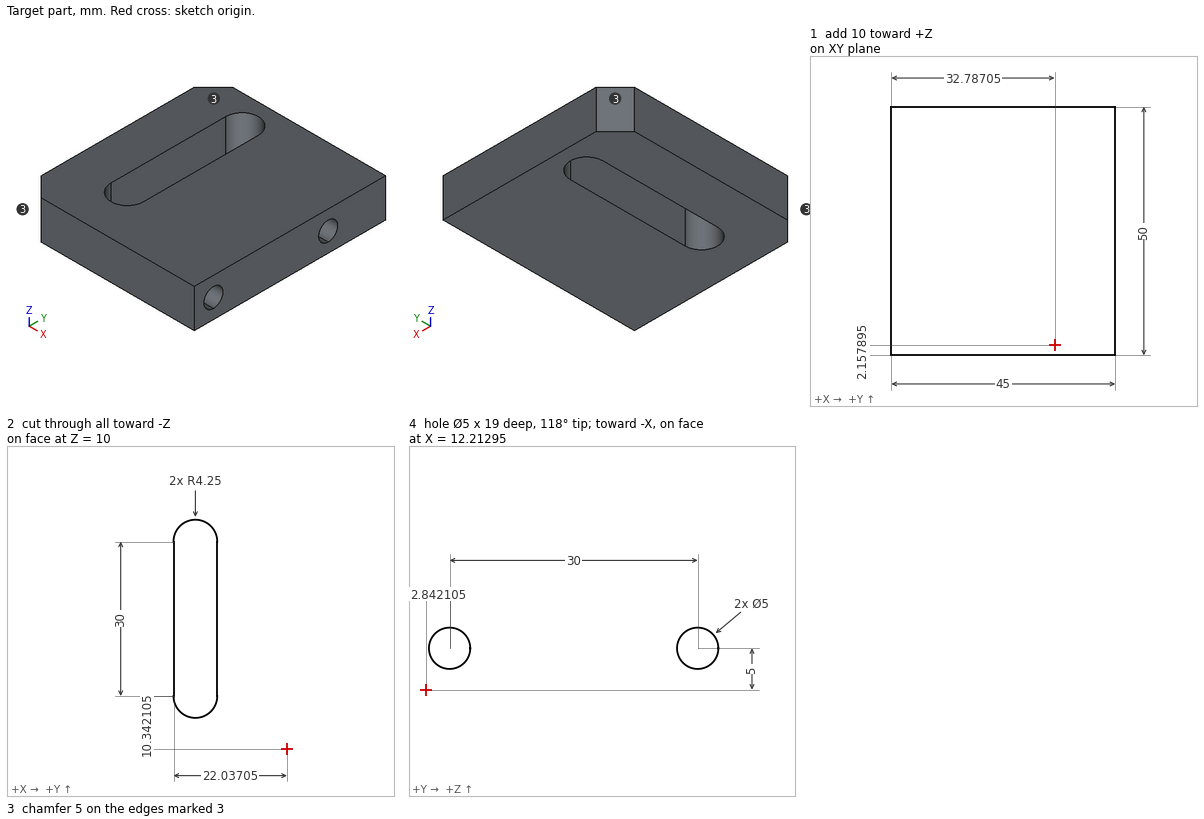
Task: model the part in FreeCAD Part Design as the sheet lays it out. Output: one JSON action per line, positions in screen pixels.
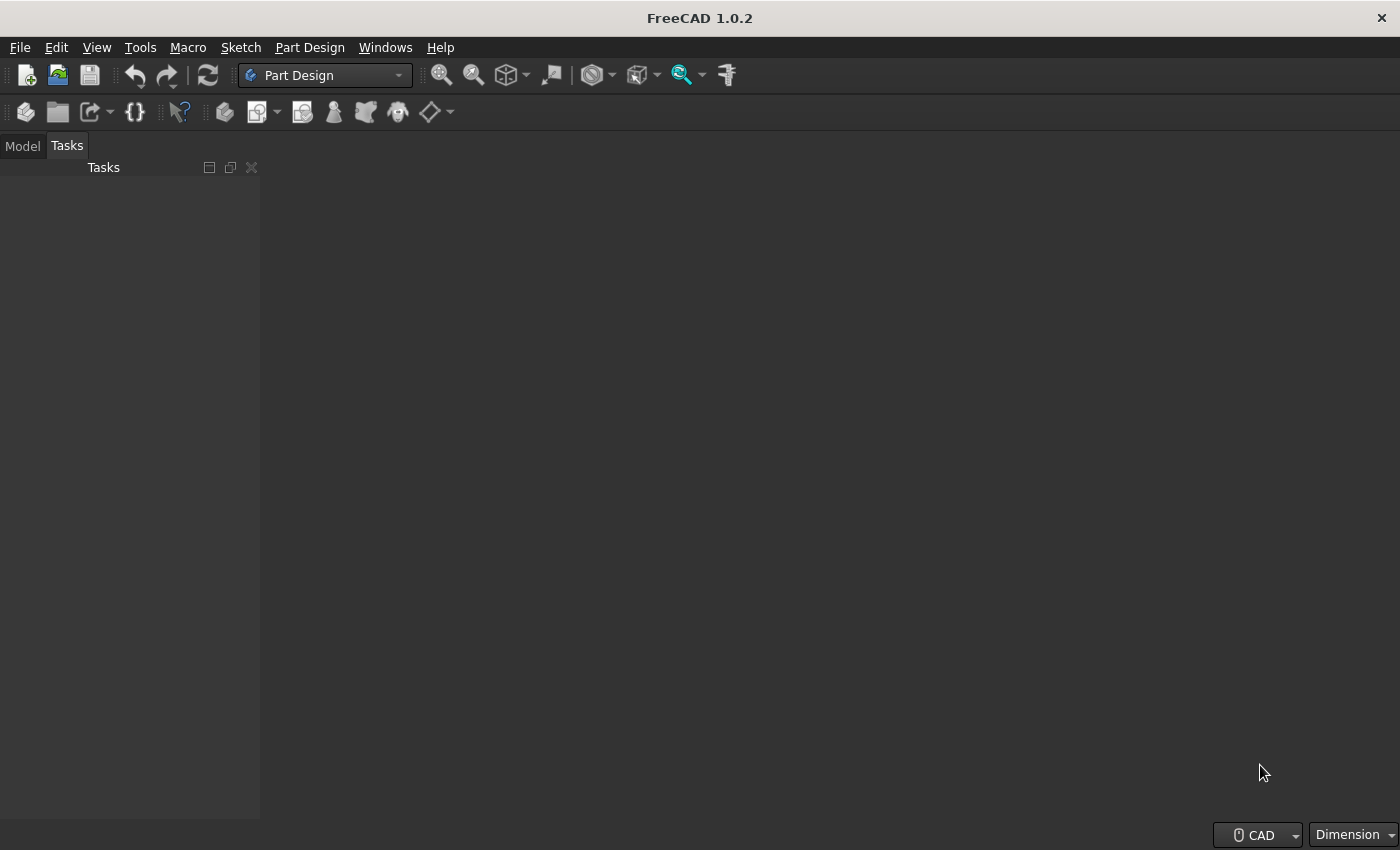
{"action": "left_click", "coordinate": [26, 76]}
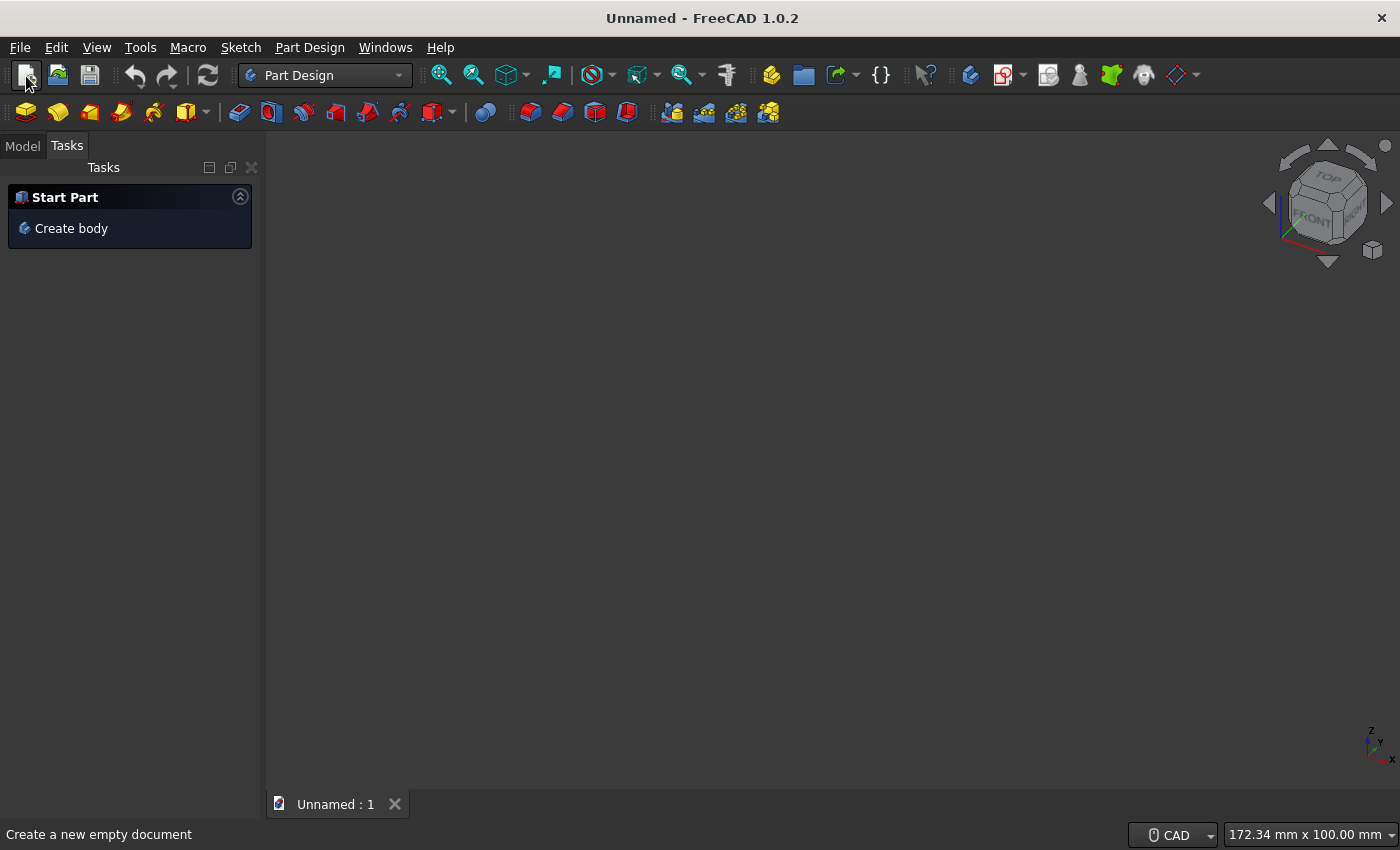
{"action": "left_click", "coordinate": [1004, 76]}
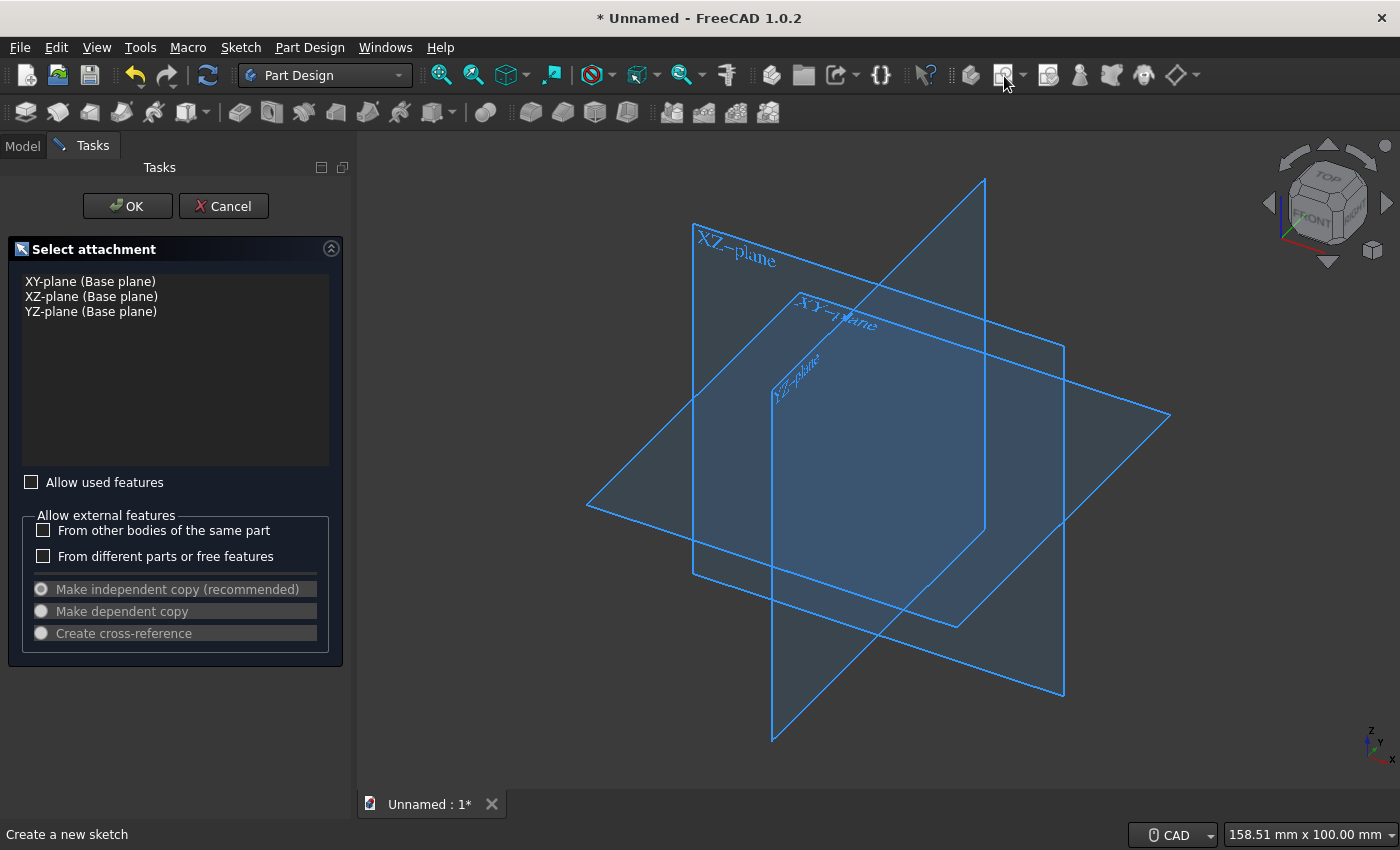
{"action": "left_click", "coordinate": [82, 282]}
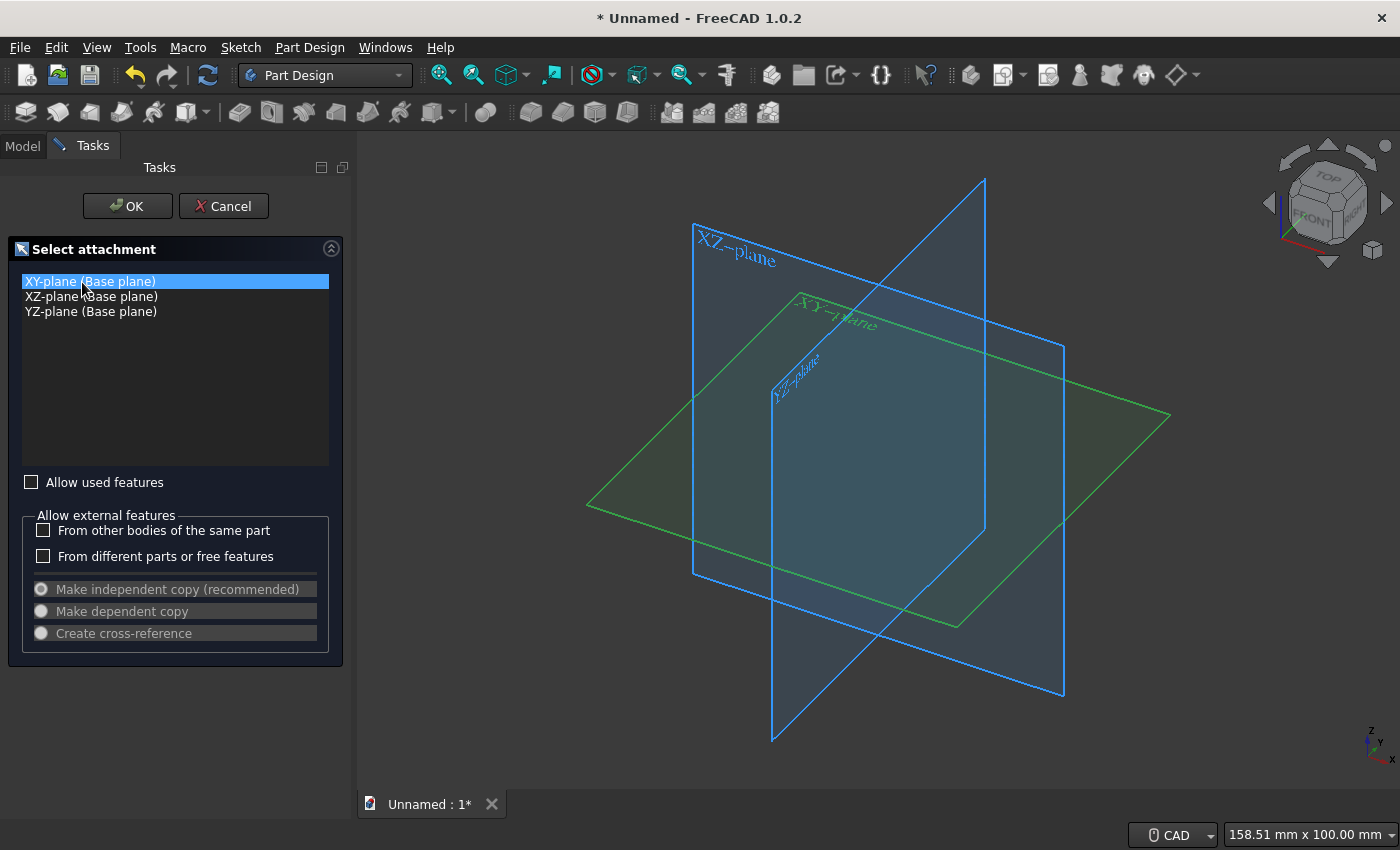
{"action": "left_click", "coordinate": [128, 206]}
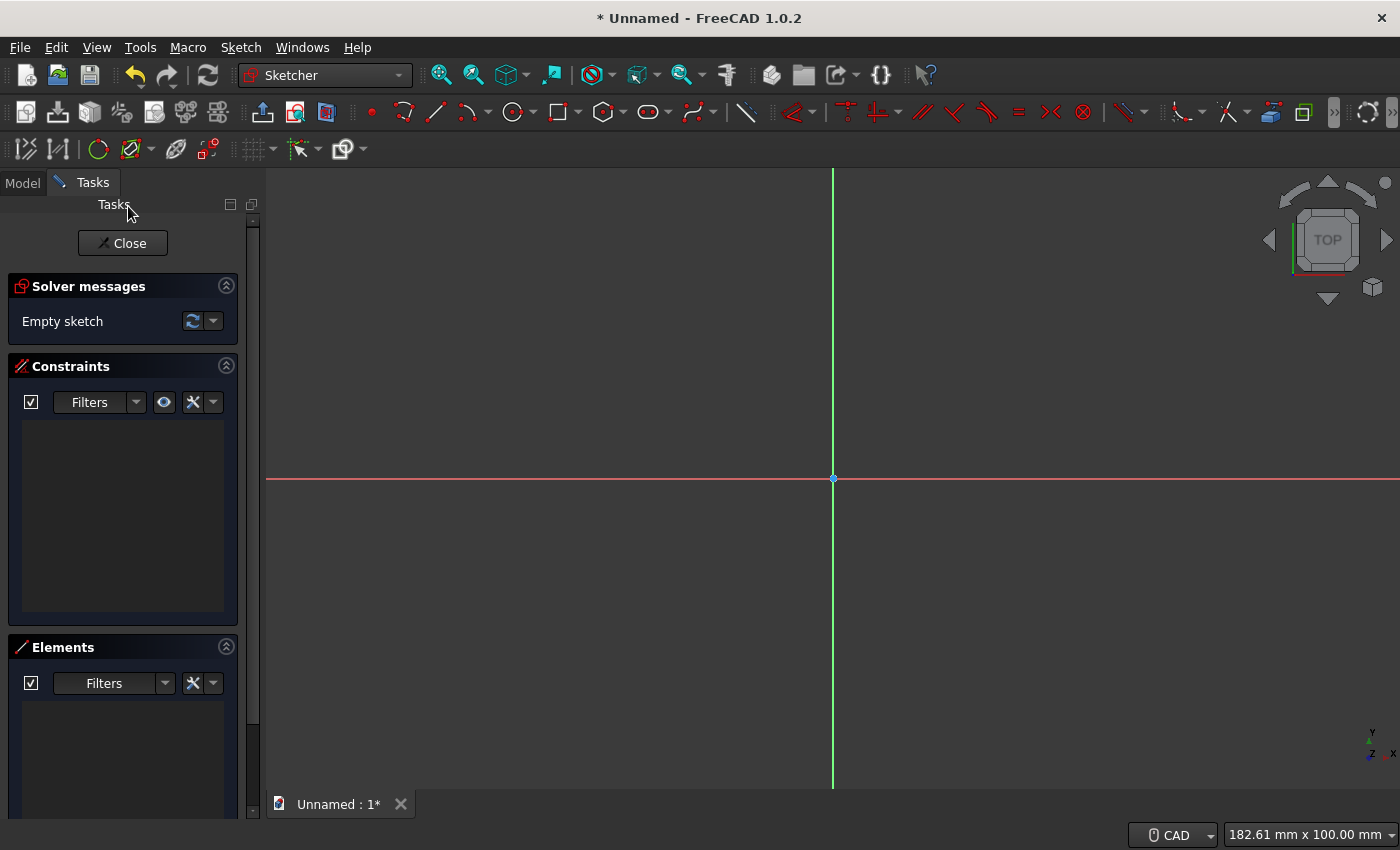
{"action": "scroll", "coordinate": [744, 761], "scroll_direction": "down", "scroll_amount": 1}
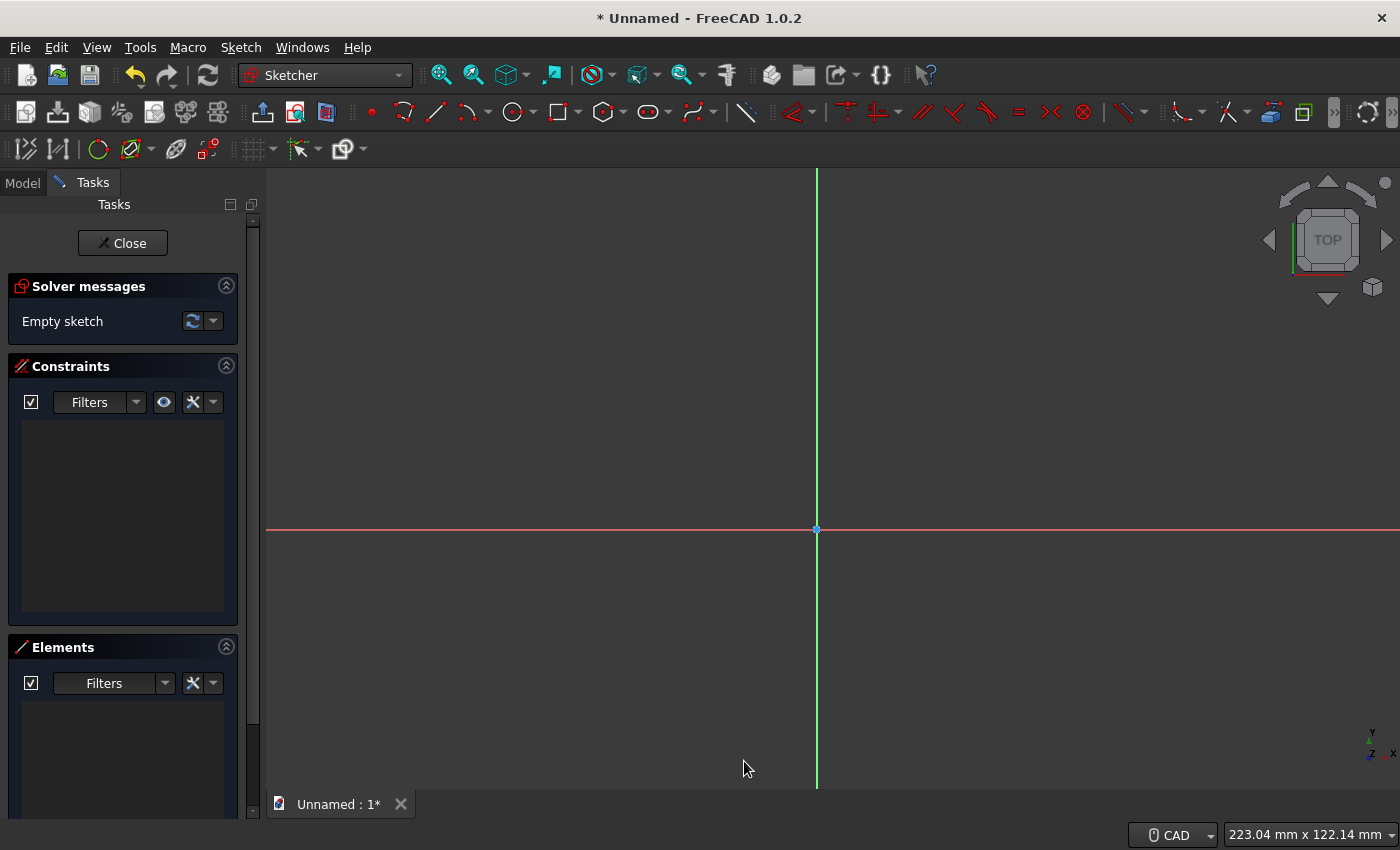
{"action": "scroll", "coordinate": [765, 282], "scroll_direction": "up", "scroll_amount": 2}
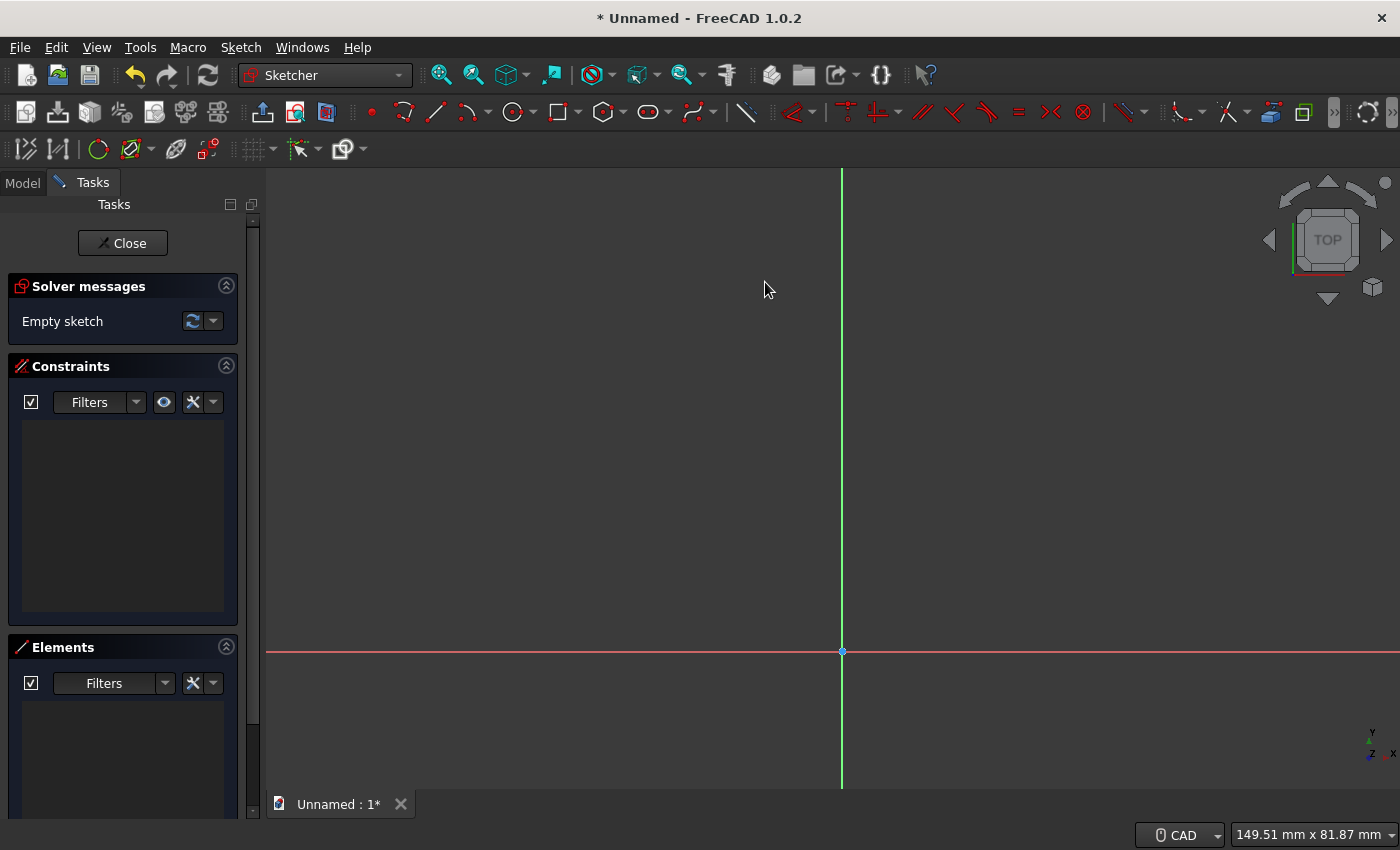
{"action": "left_click", "coordinate": [558, 112]}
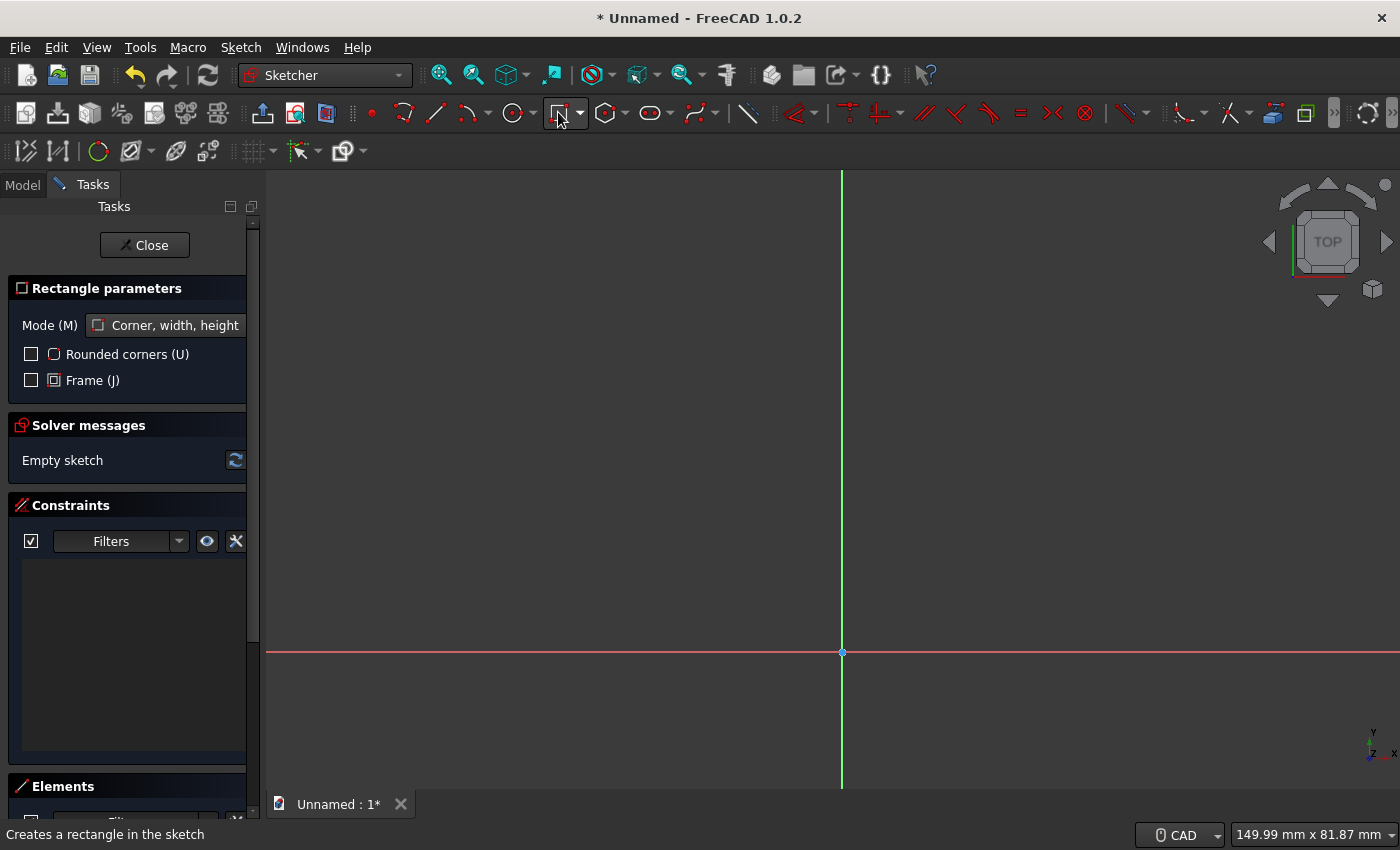
{"action": "left_click", "coordinate": [594, 290]}
{"action": "mouse_move", "coordinate": [935, 668]}